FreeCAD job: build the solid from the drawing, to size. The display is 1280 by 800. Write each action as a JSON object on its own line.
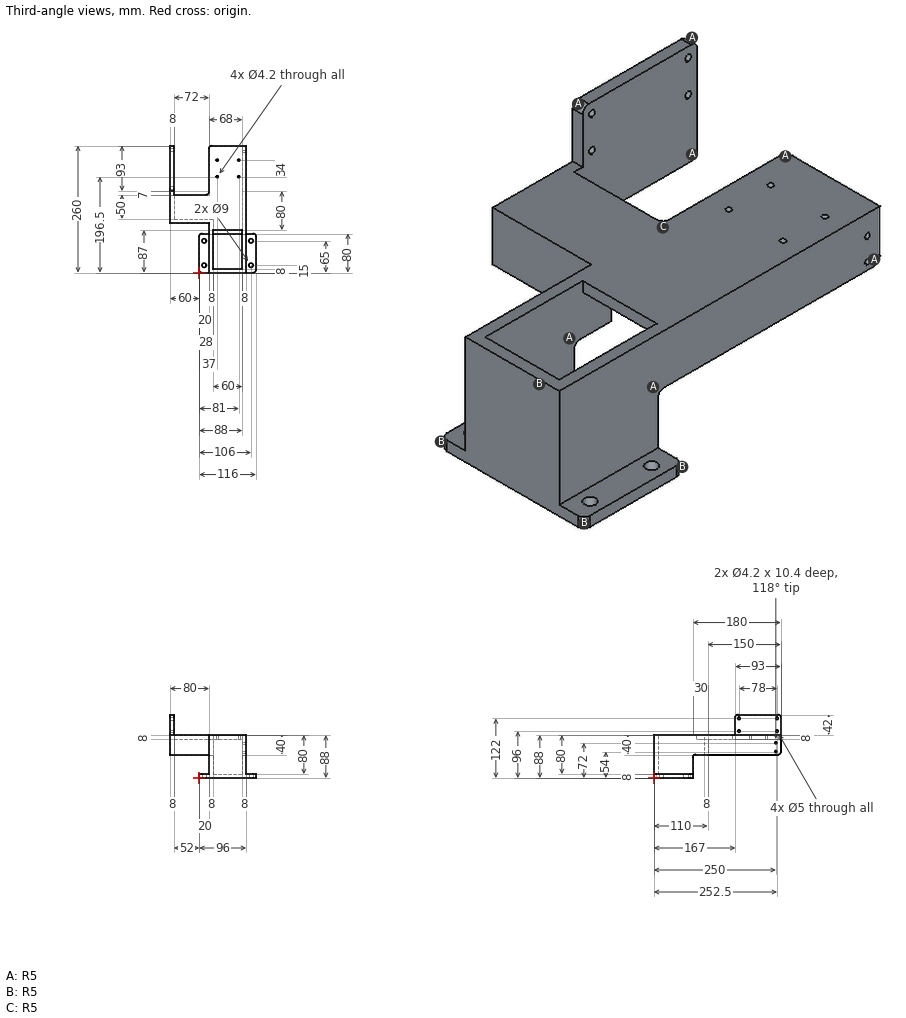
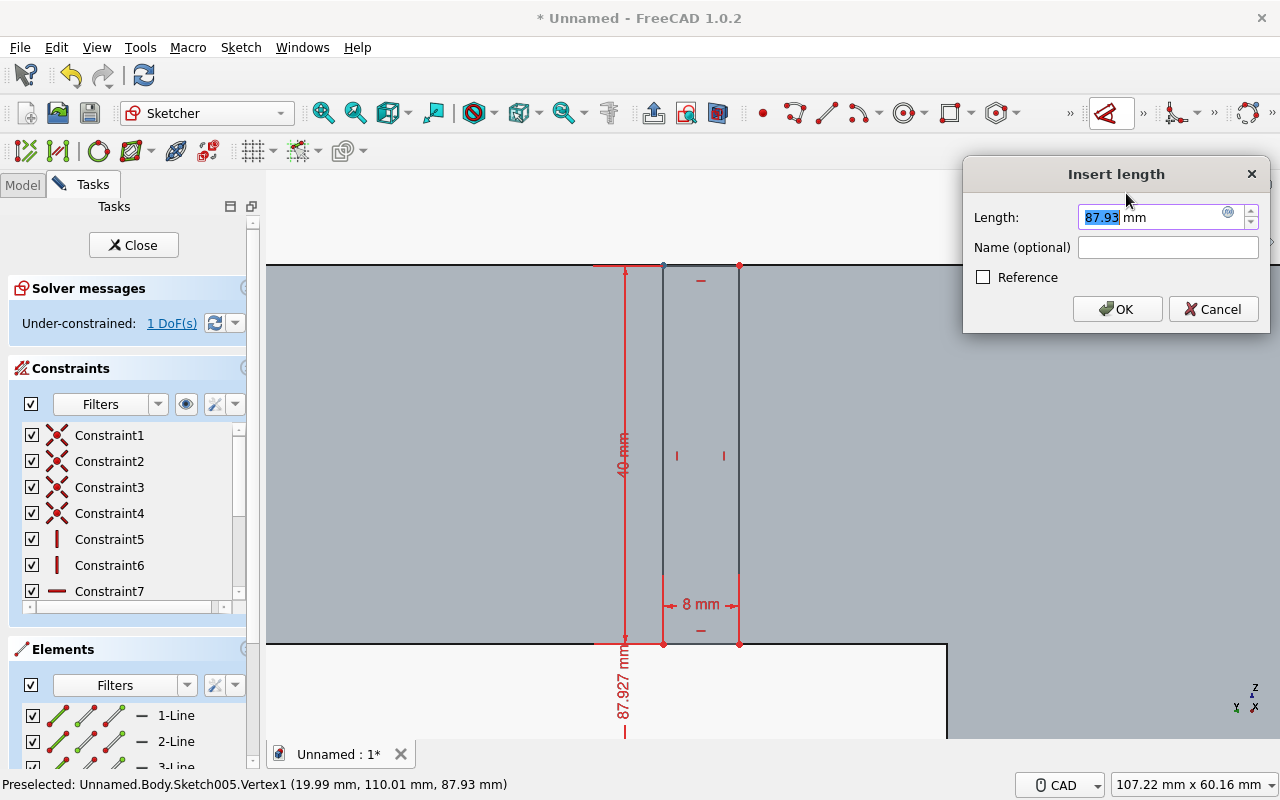
{"action": "type", "text": "88"}
{"action": "key", "text": "Return"}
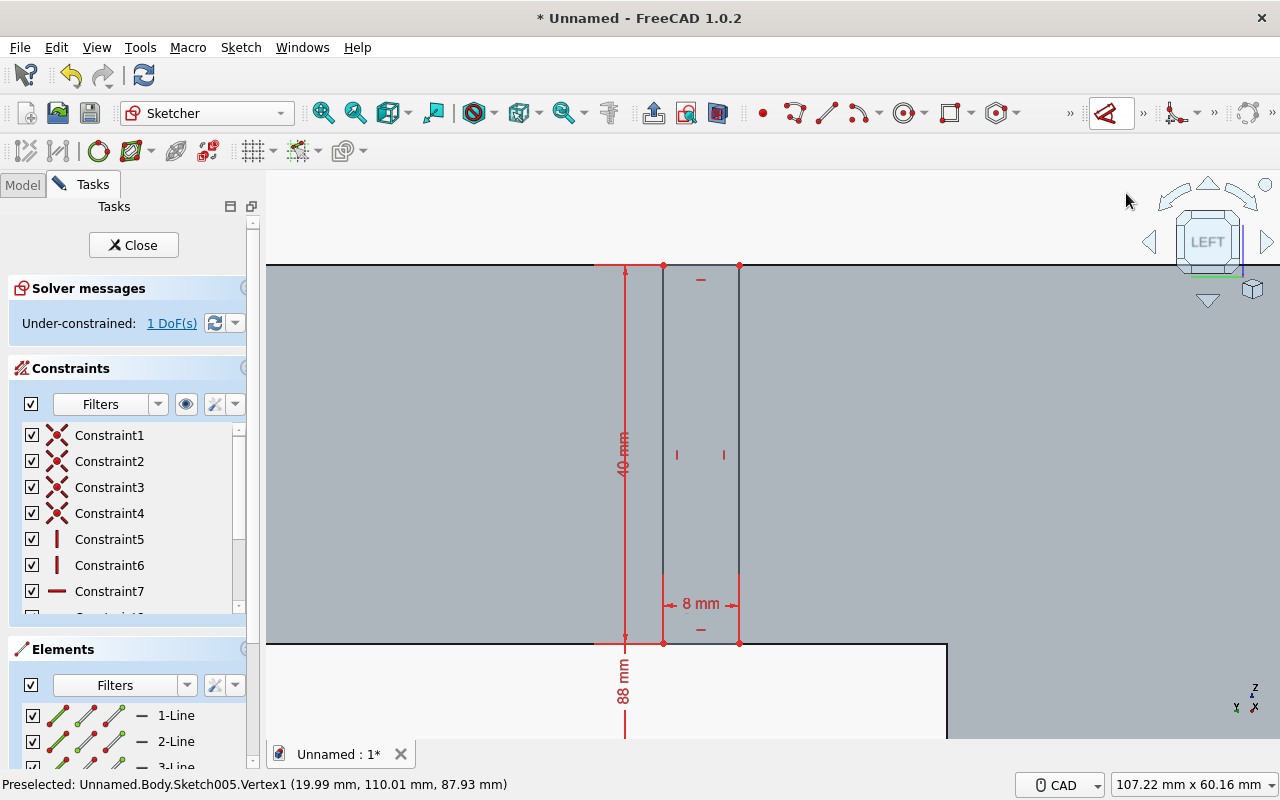
{"action": "left_click", "coordinate": [663, 265]}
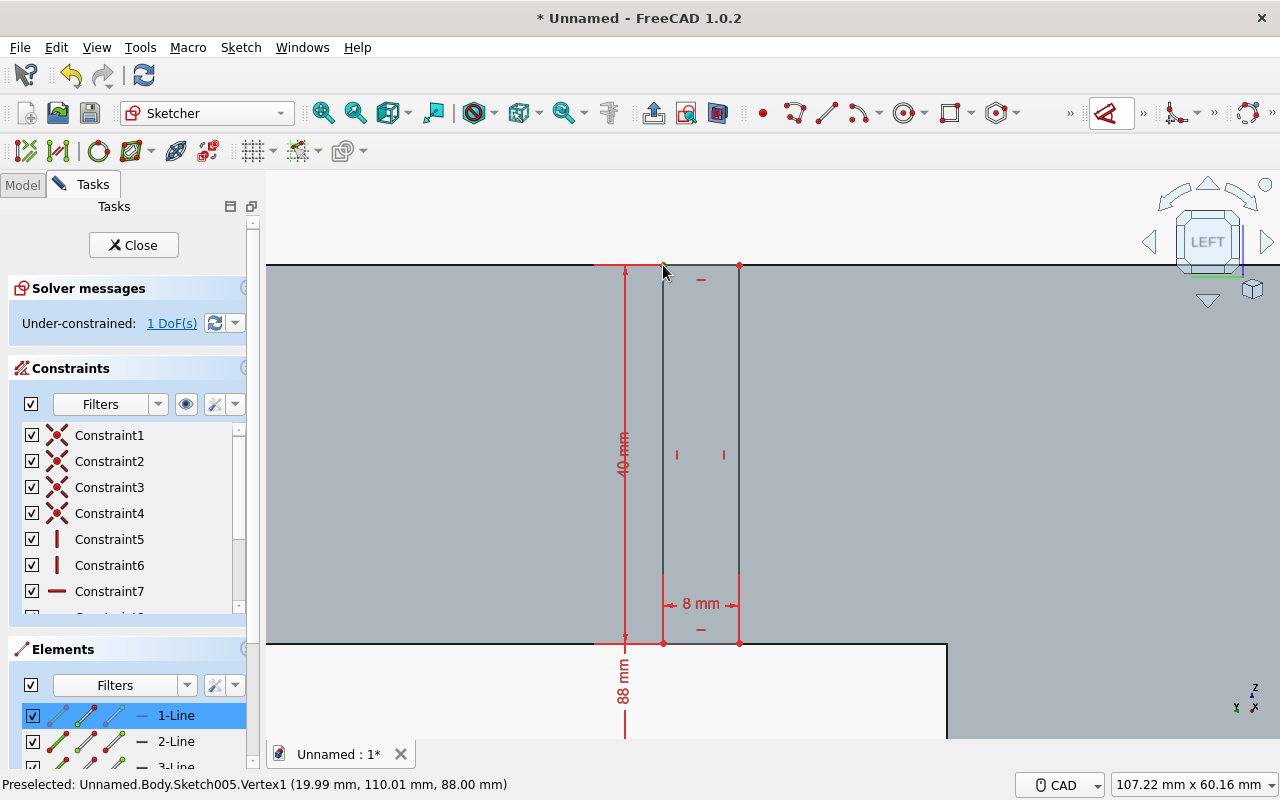
{"action": "left_click", "coordinate": [1128, 114]}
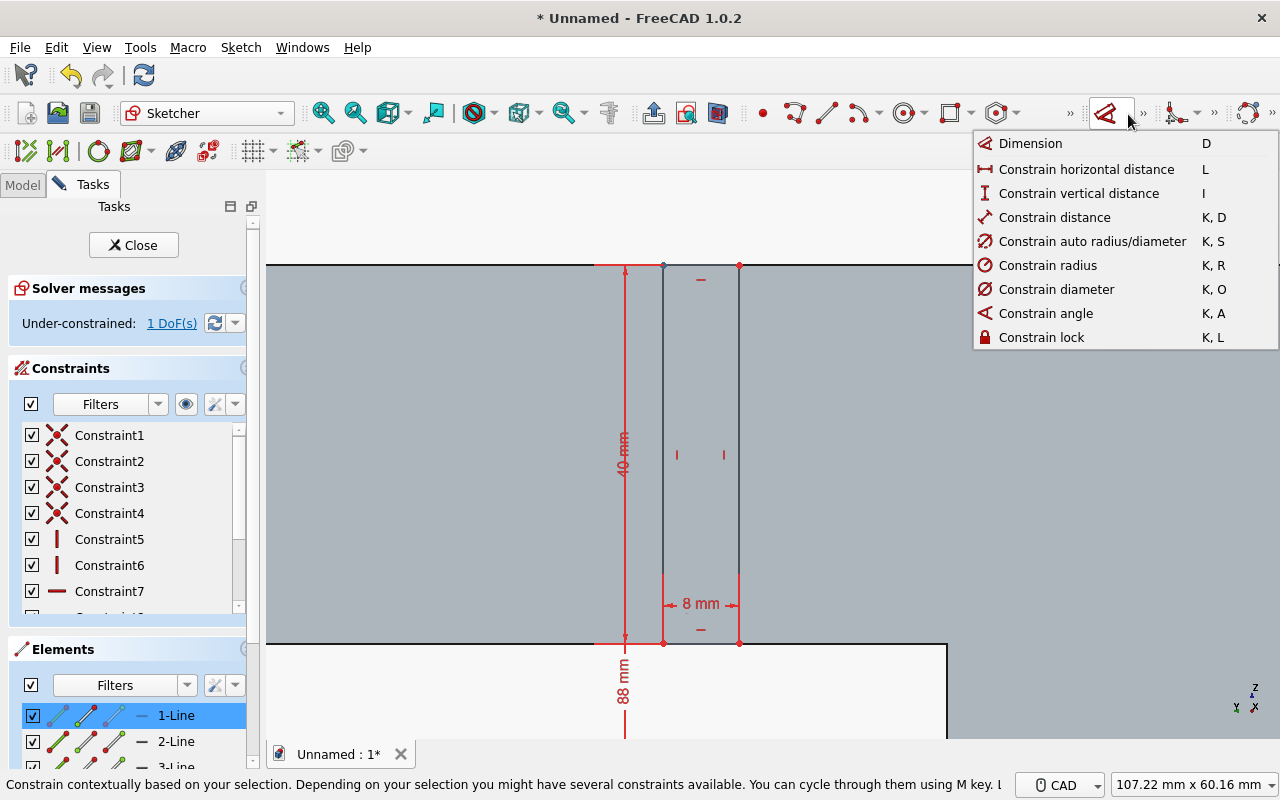
{"action": "left_click", "coordinate": [1126, 169]}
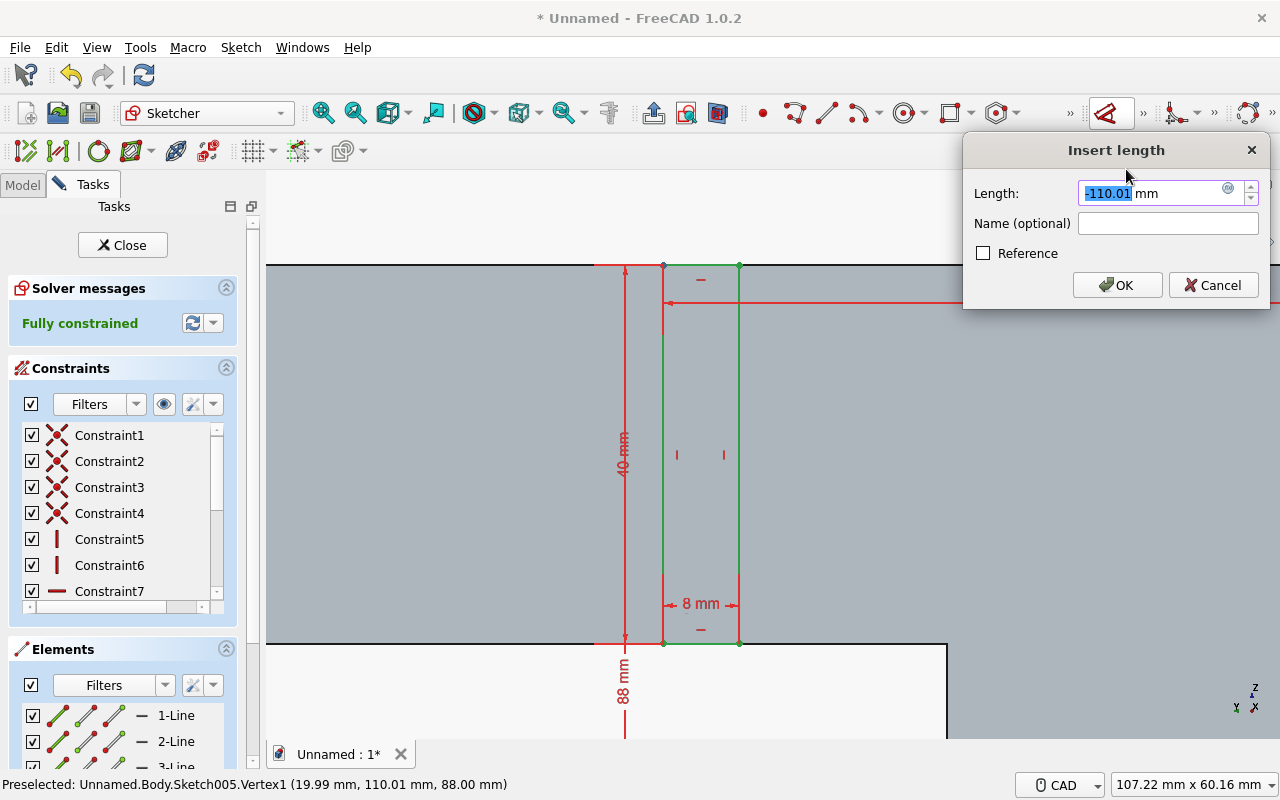
{"action": "type", "text": "-110"}
{"action": "key", "text": "Return"}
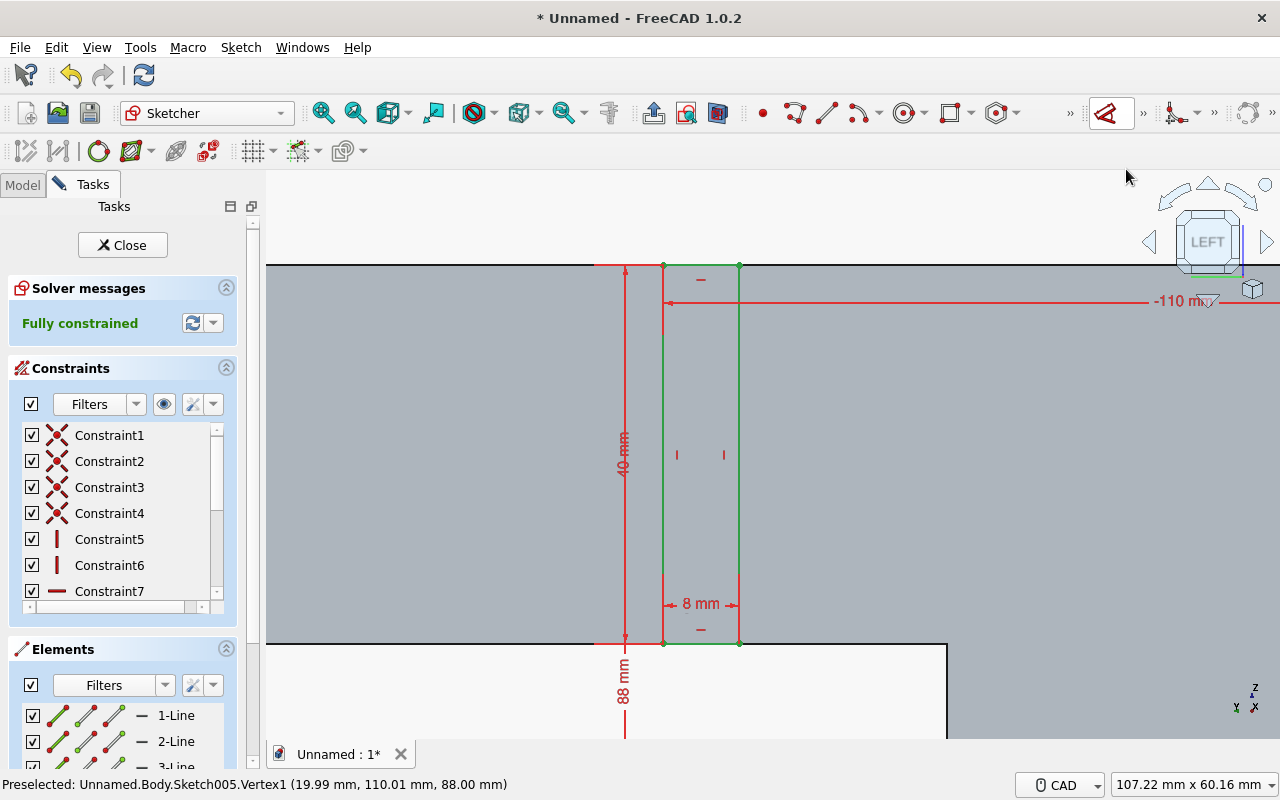
{"action": "left_click", "coordinate": [123, 245]}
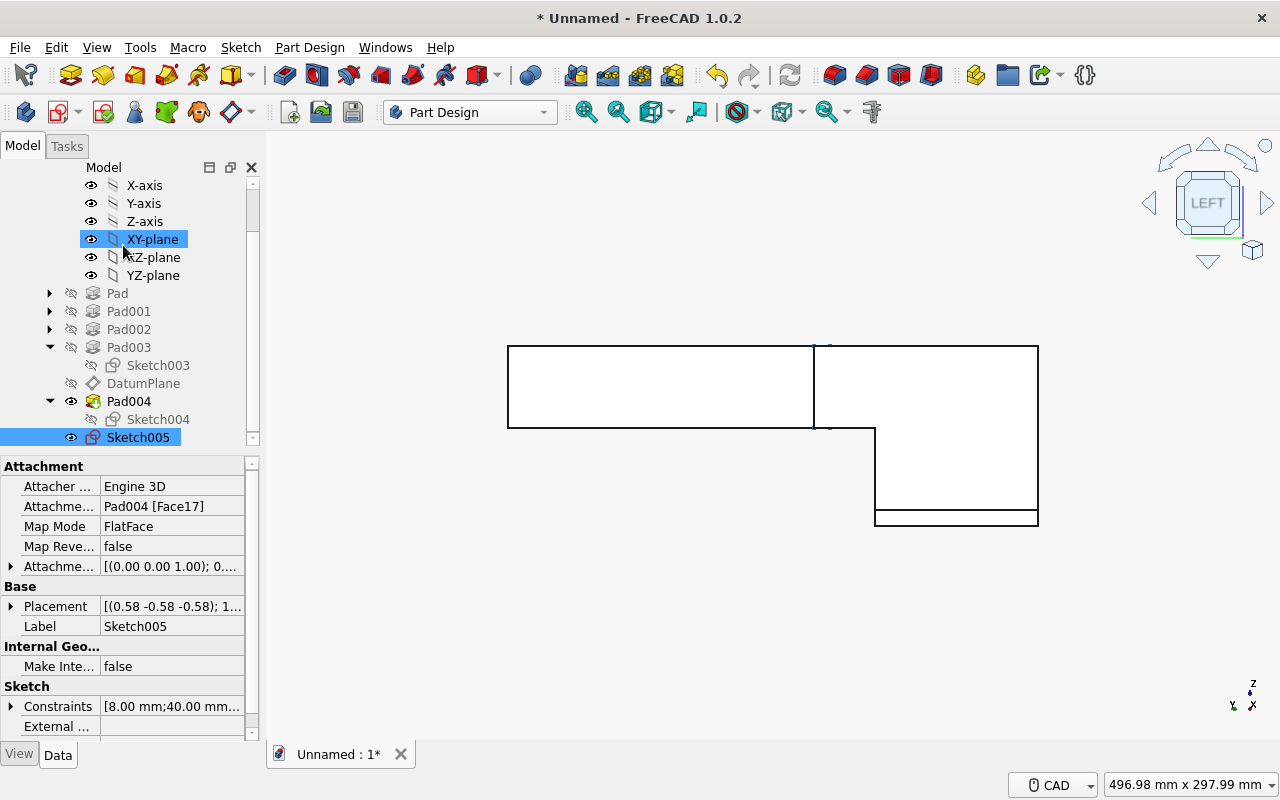
{"action": "left_click", "coordinate": [72, 76]}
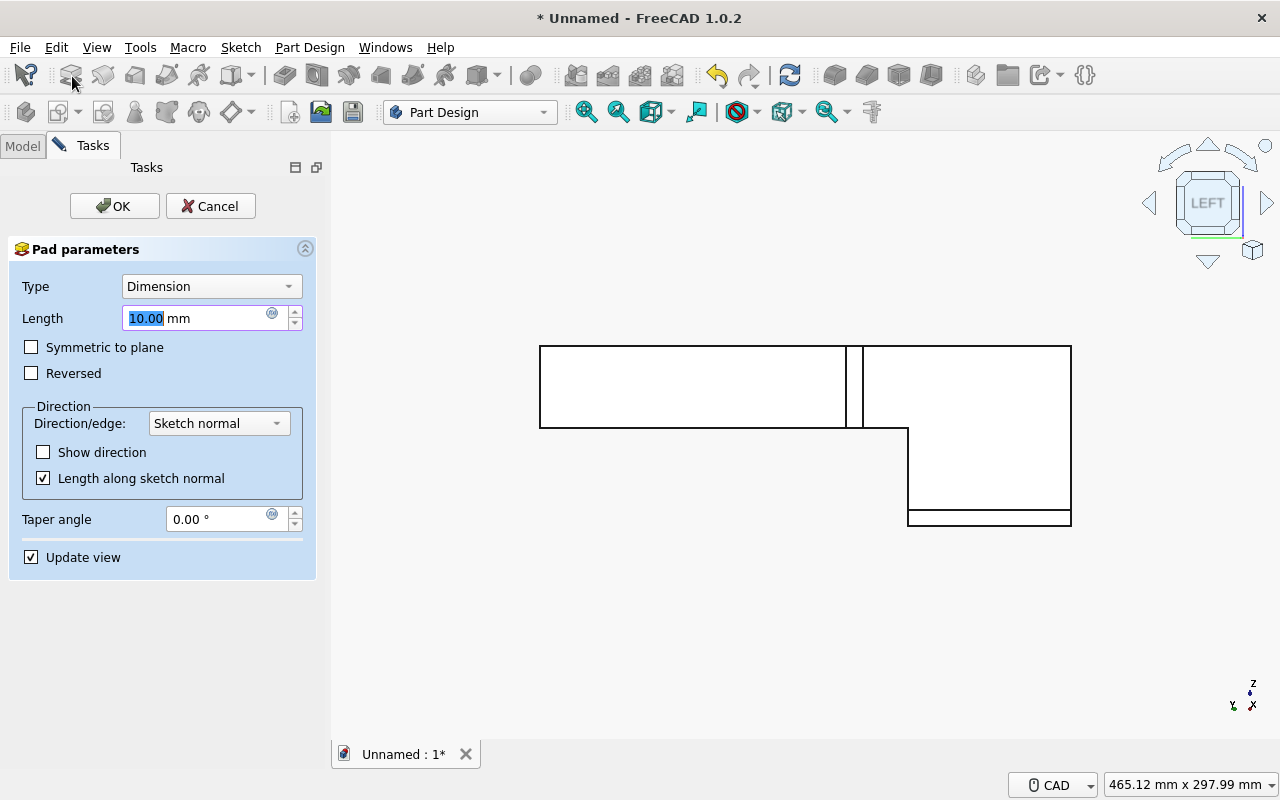
{"action": "type", "text": "80"}
{"action": "key", "text": "Tab"}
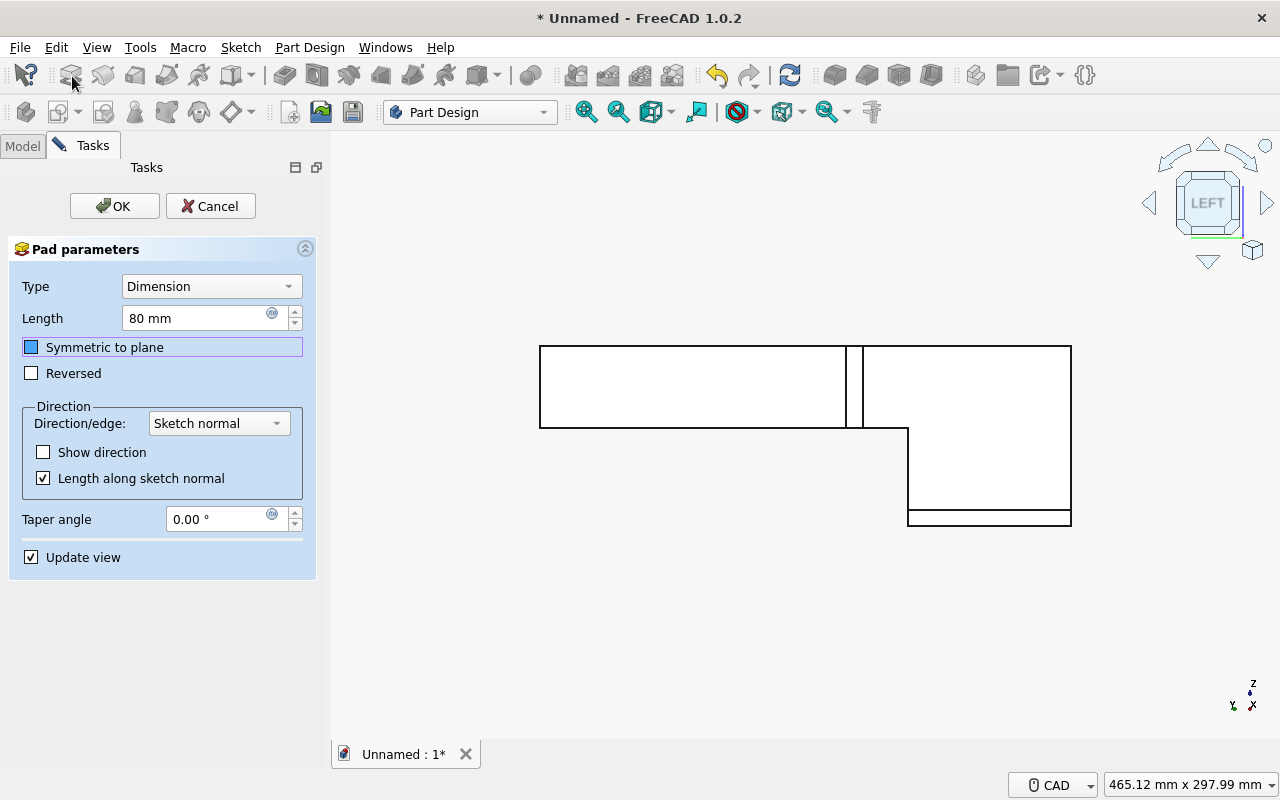
{"action": "left_click", "coordinate": [115, 206]}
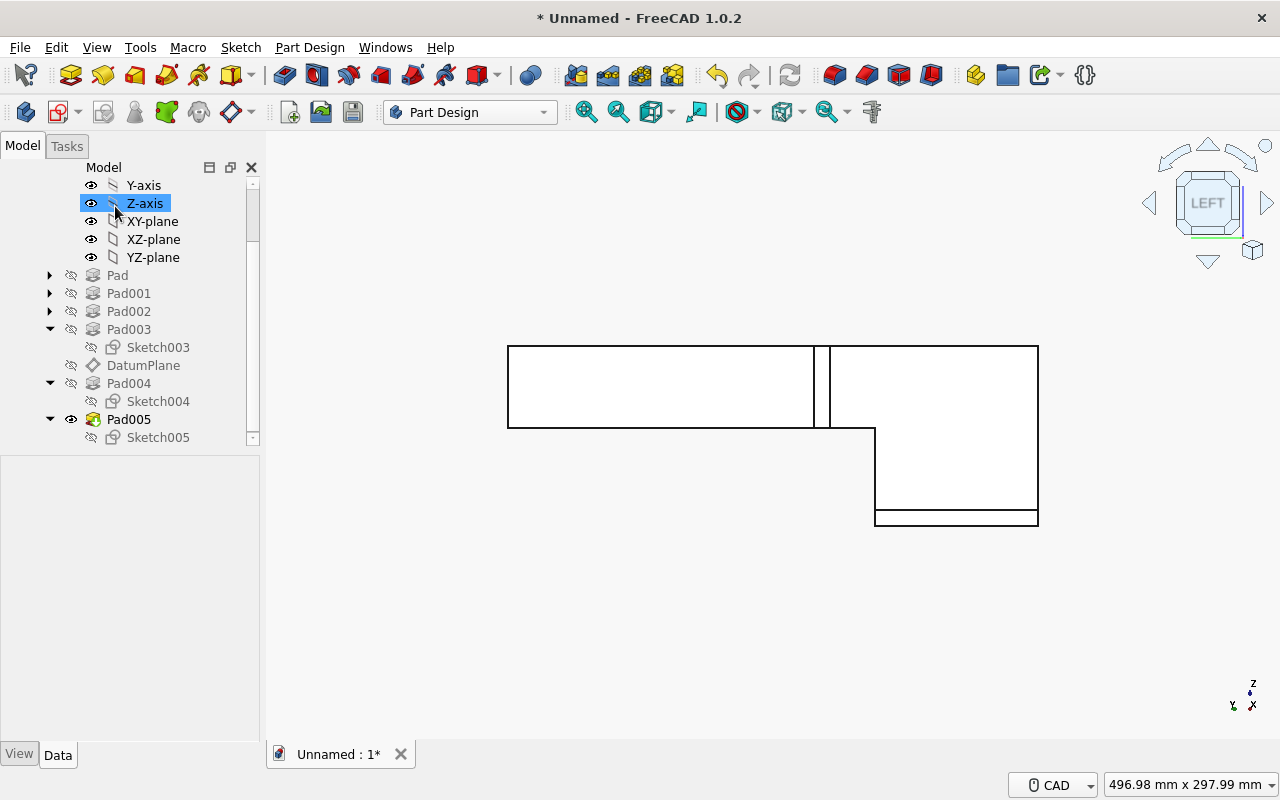
{"action": "key", "text": "4"}